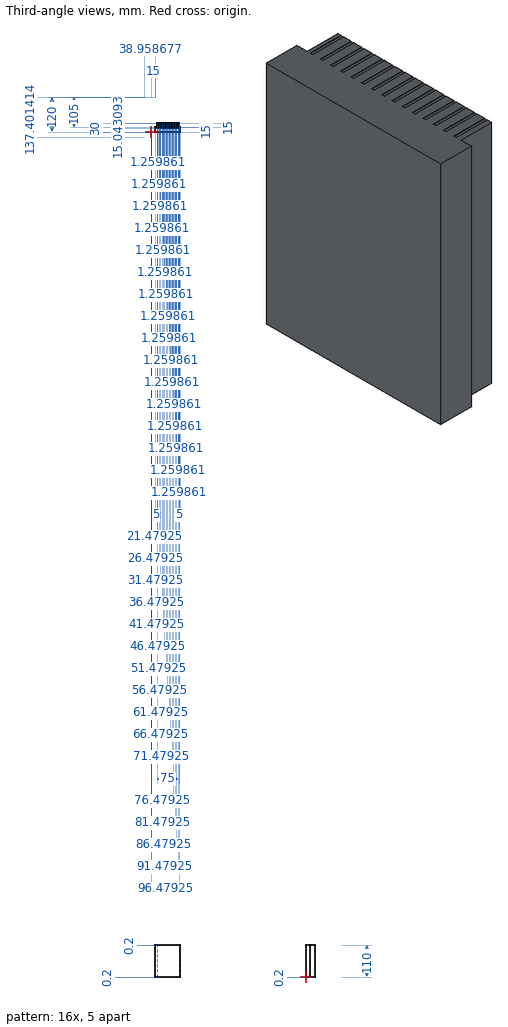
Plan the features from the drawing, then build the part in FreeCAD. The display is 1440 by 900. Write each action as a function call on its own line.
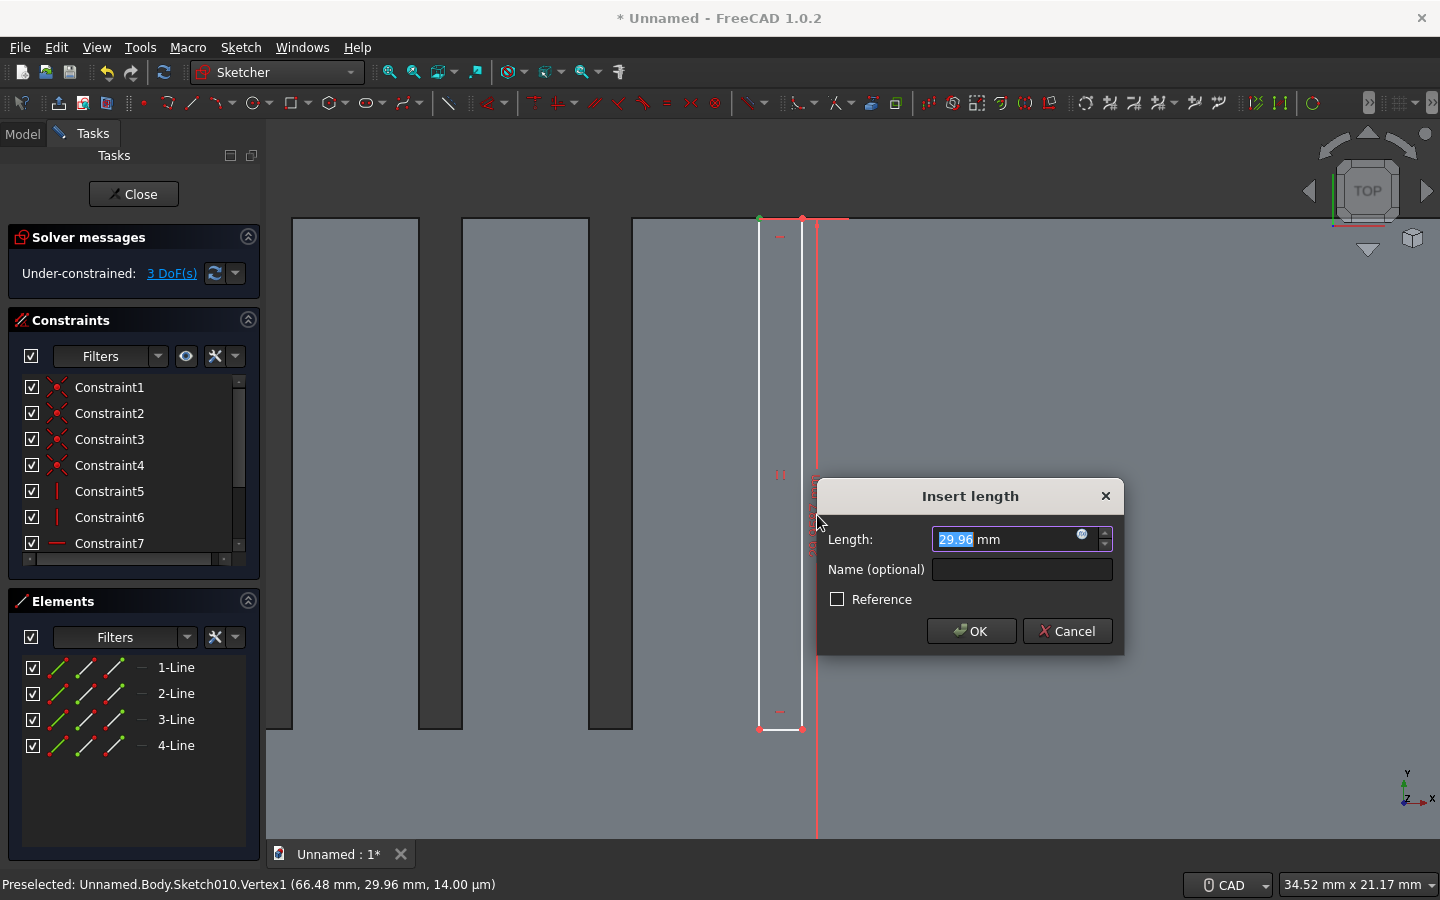
text(30)
key(Return)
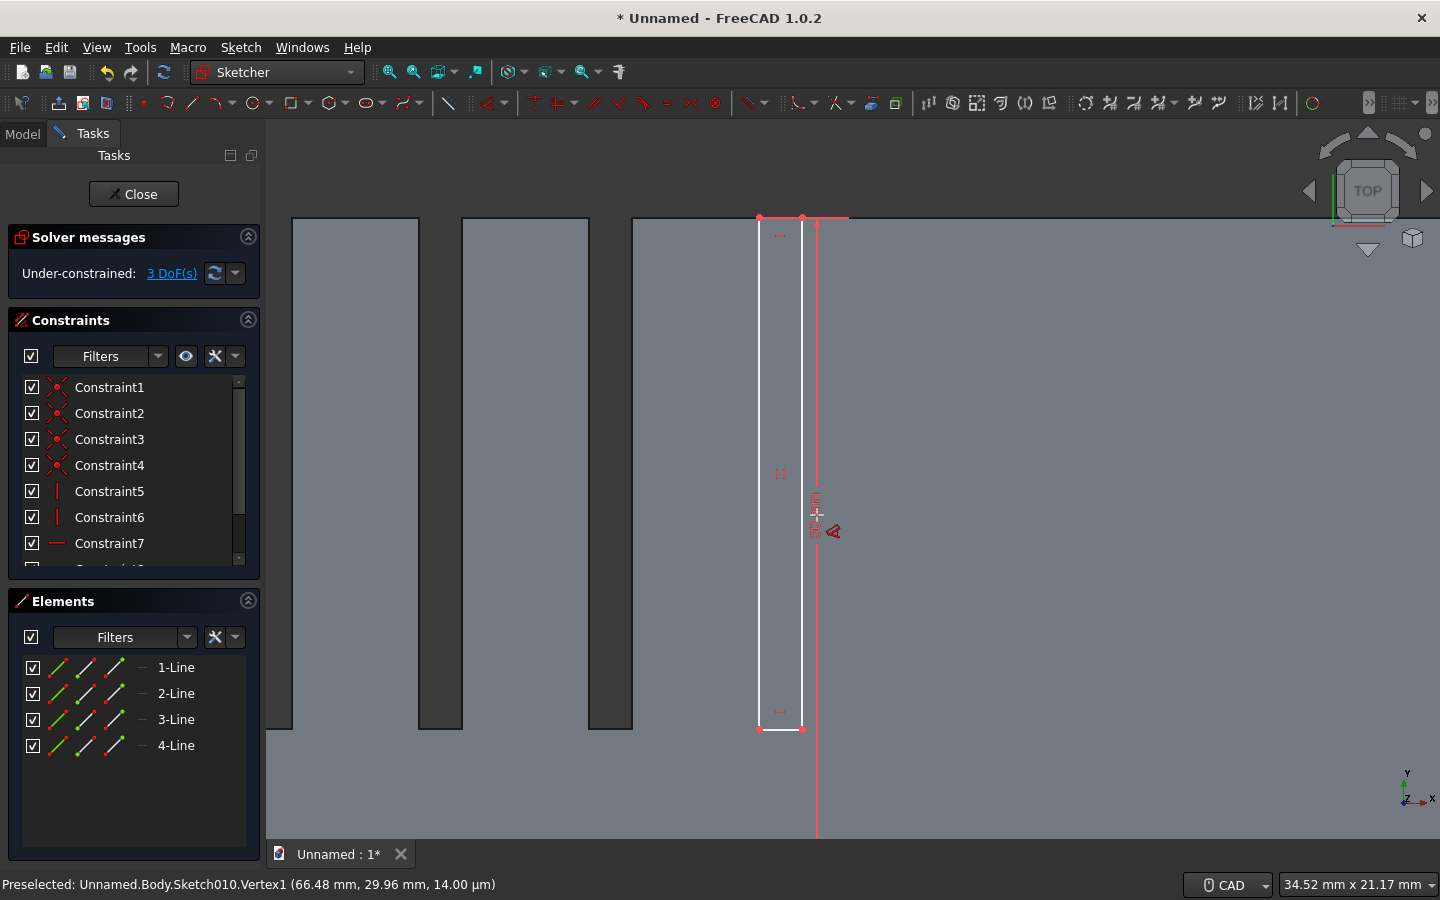
click(772, 730)
click(781, 764)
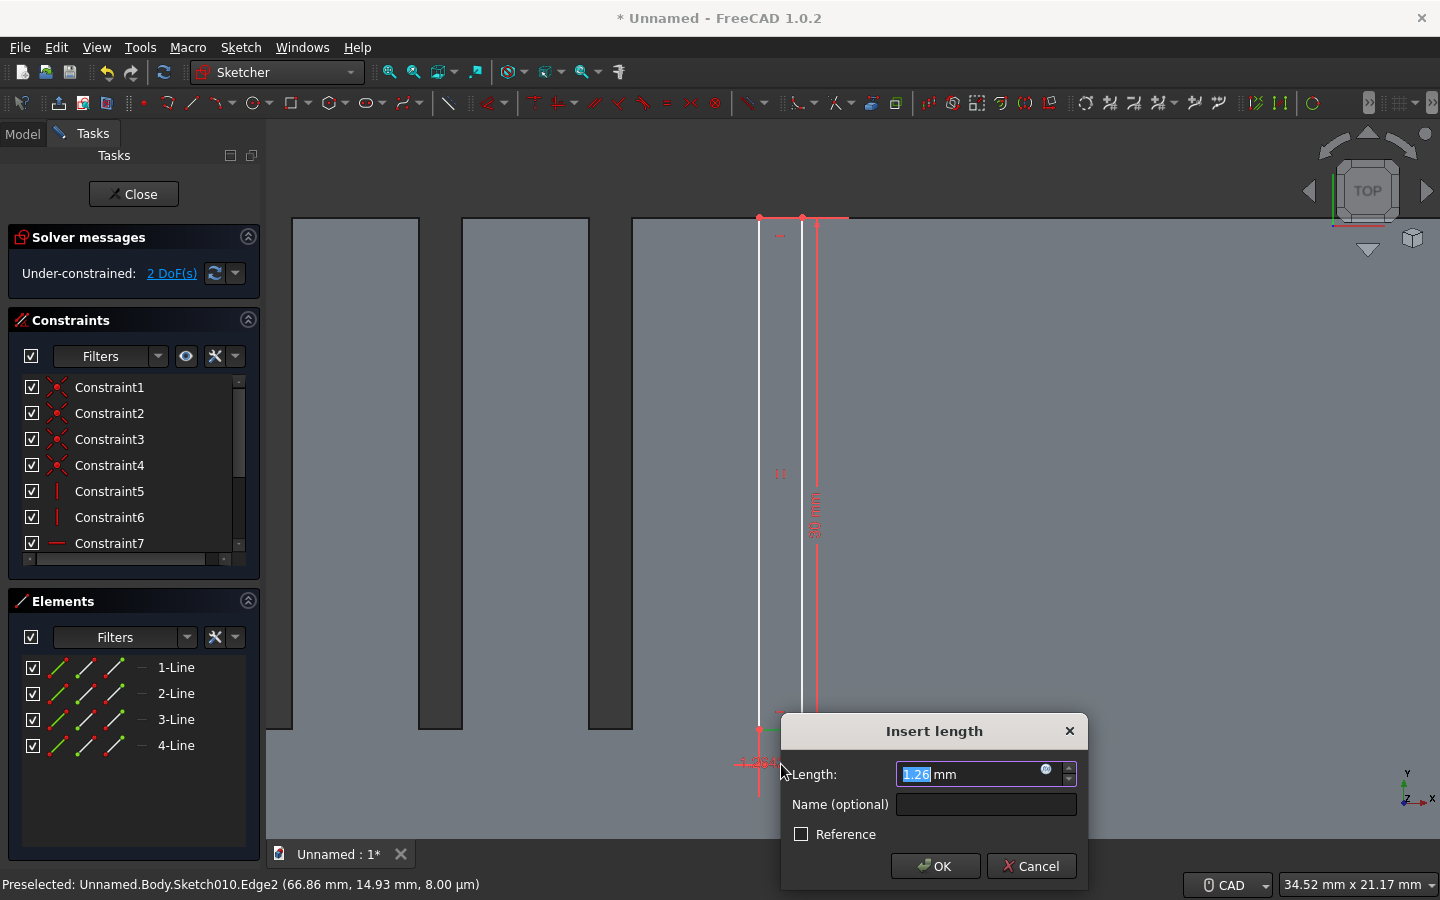
text(1.259861)
key(Return)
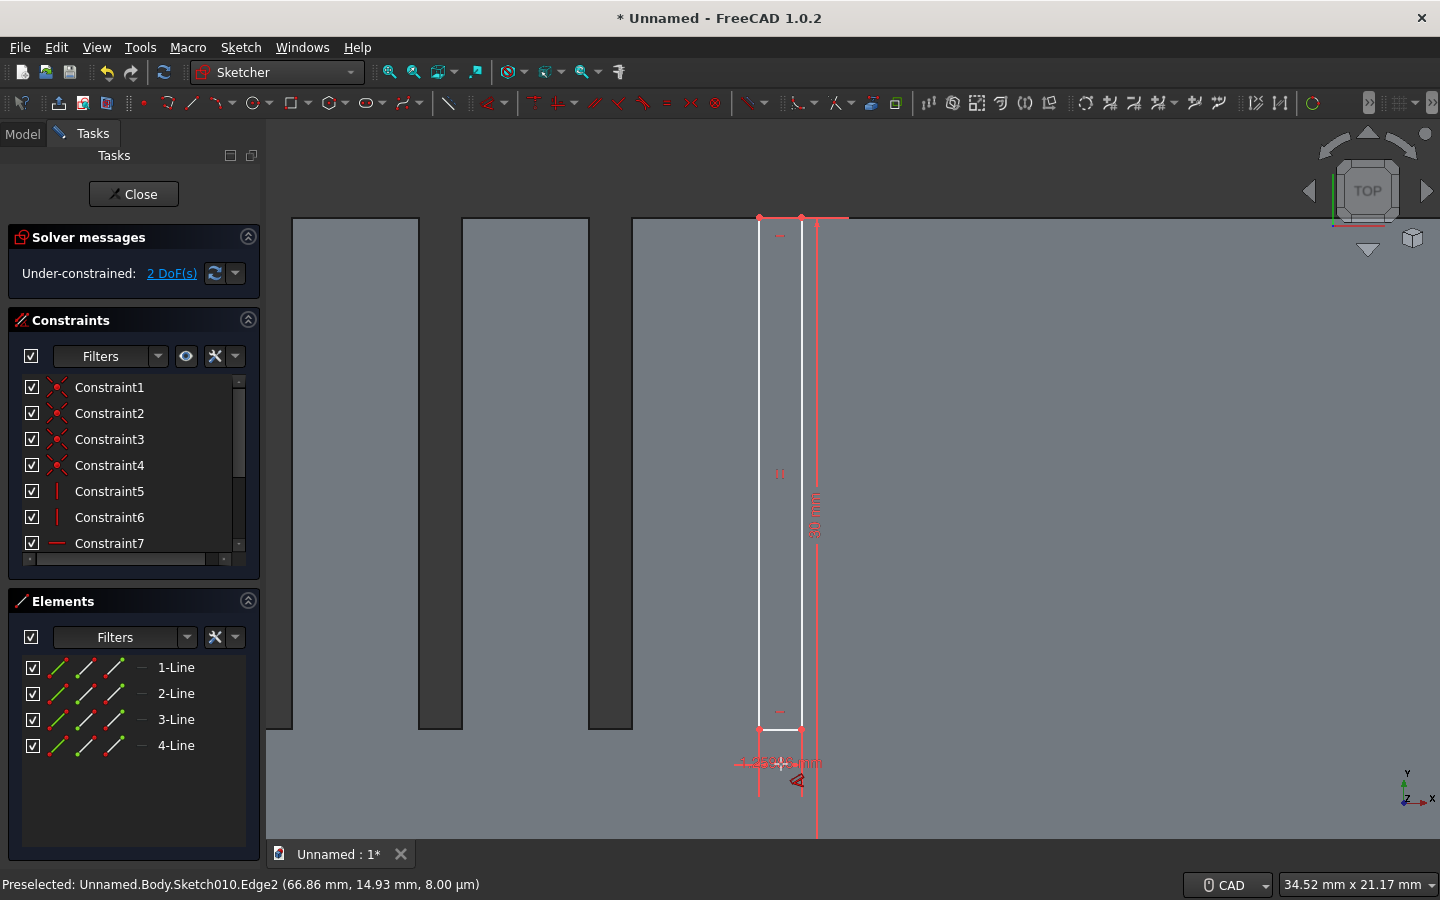
click(759, 371)
click(725, 474)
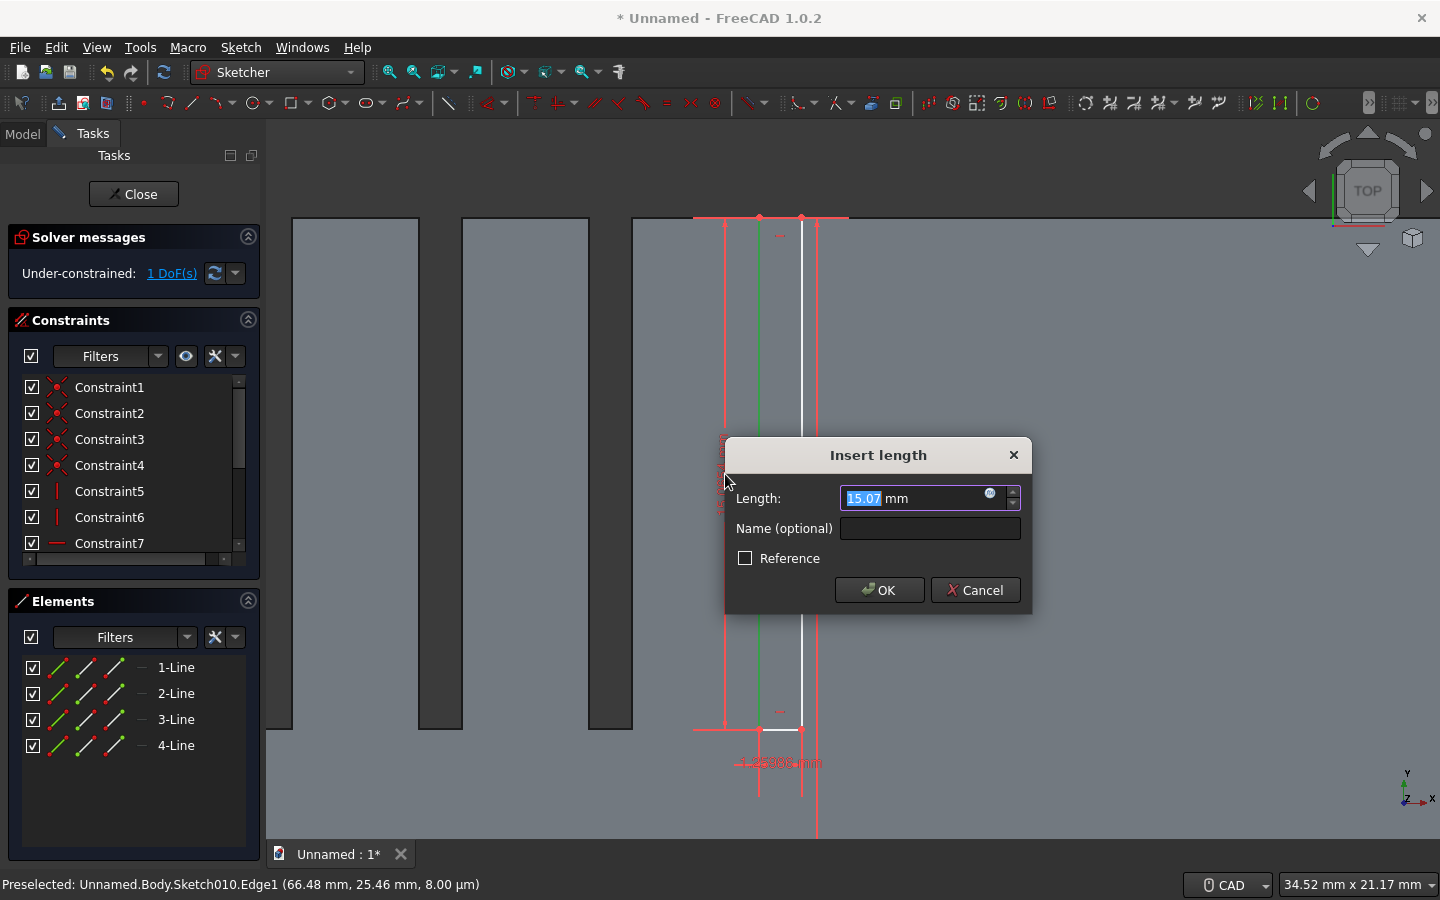
text(15.043093)
key(Return)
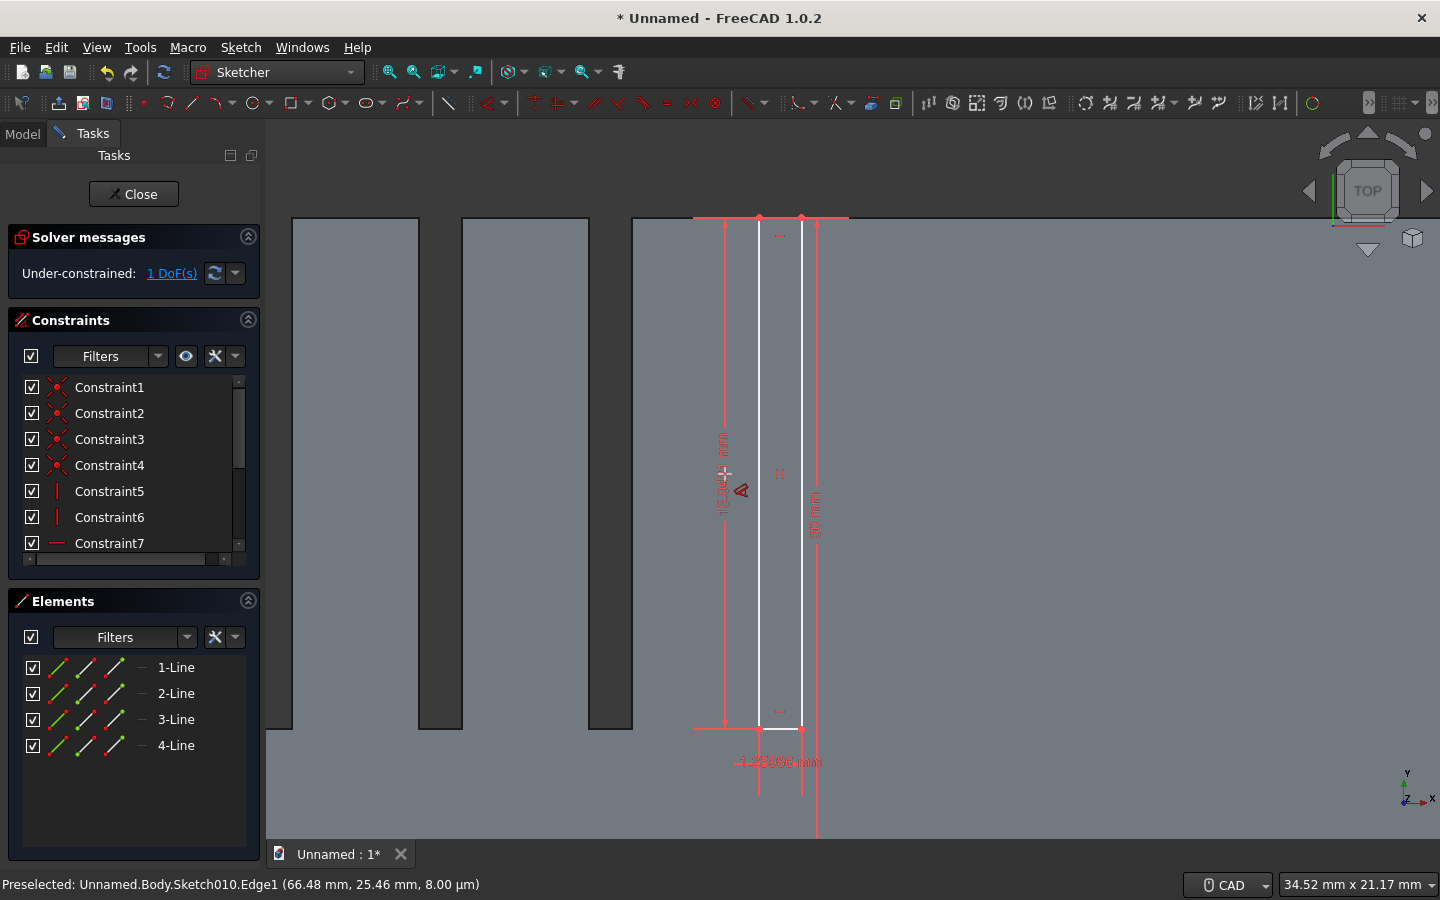
click(759, 218)
click(527, 184)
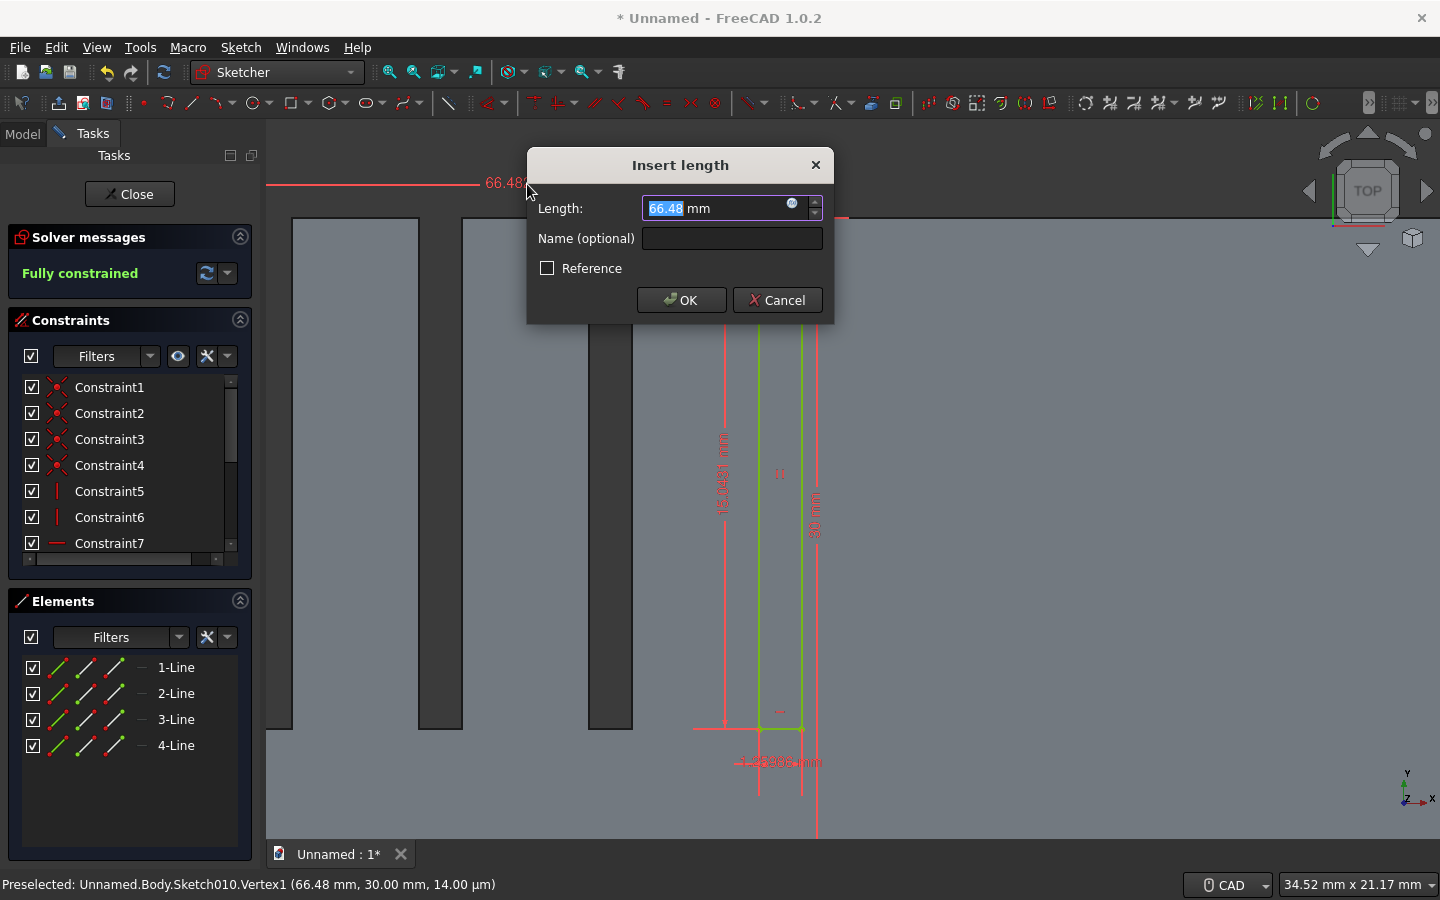
text(66.47925)
key(Return)
key(Escape)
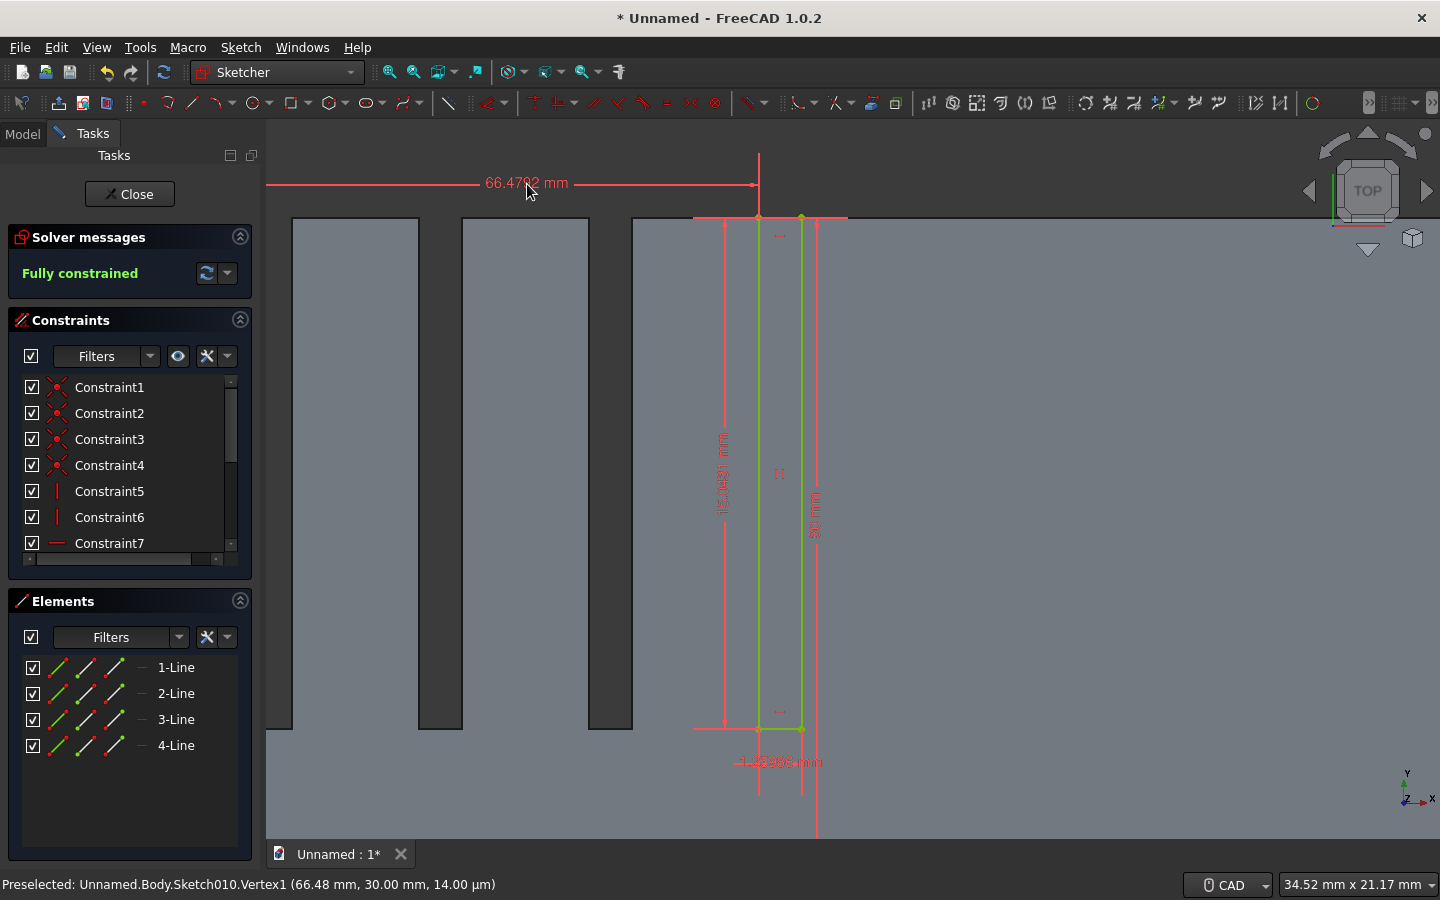
click(130, 194)